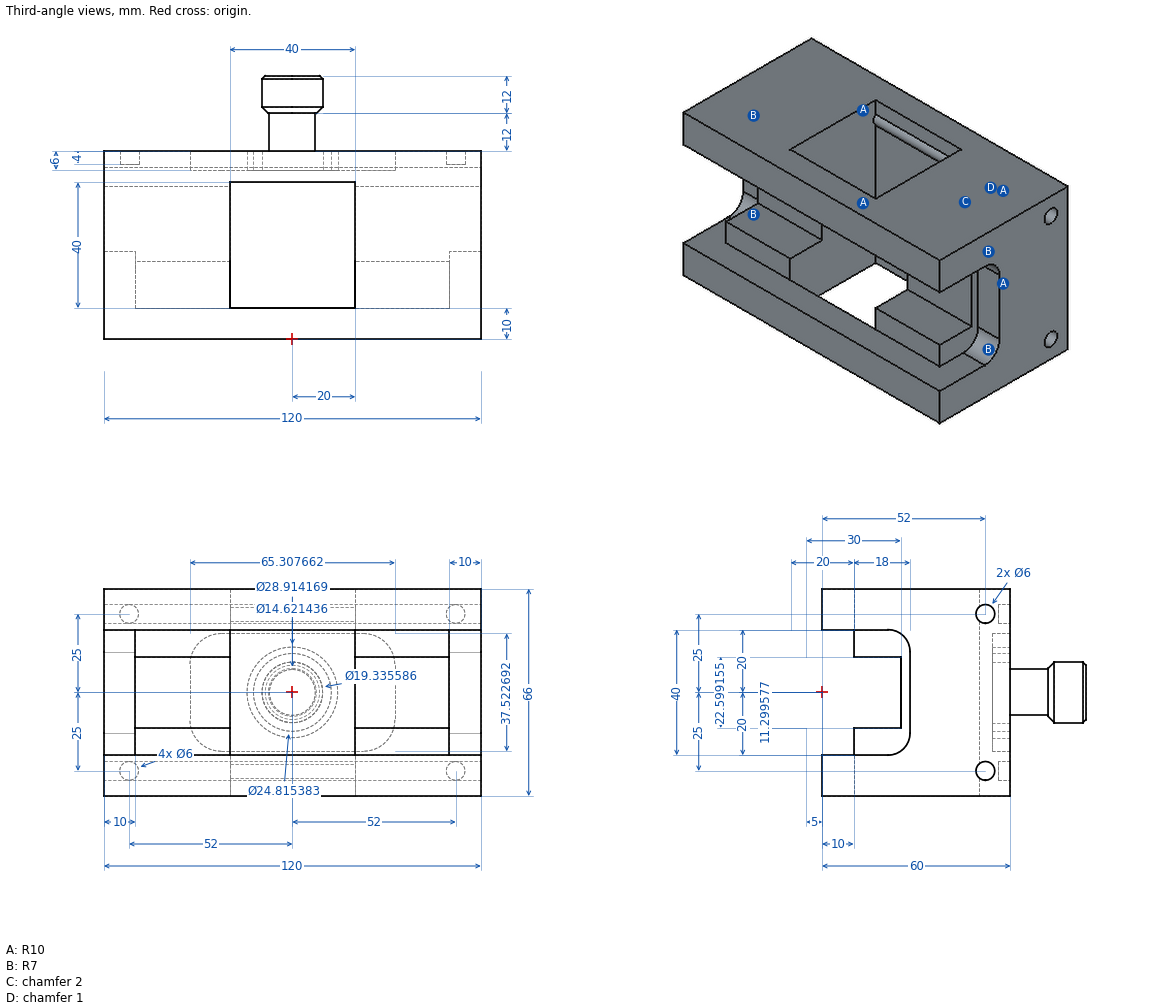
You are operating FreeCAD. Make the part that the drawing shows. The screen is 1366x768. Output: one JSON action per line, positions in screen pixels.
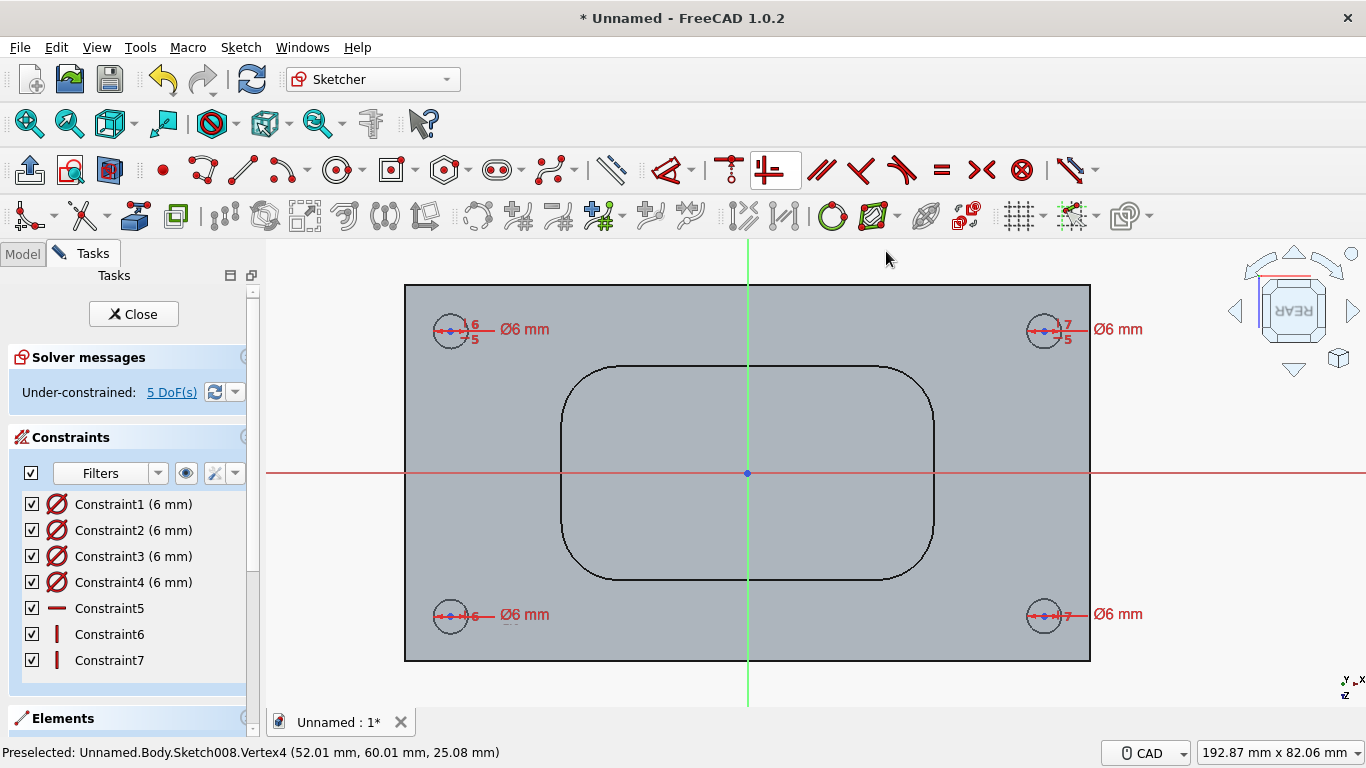
{"action": "left_click", "coordinate": [451, 617]}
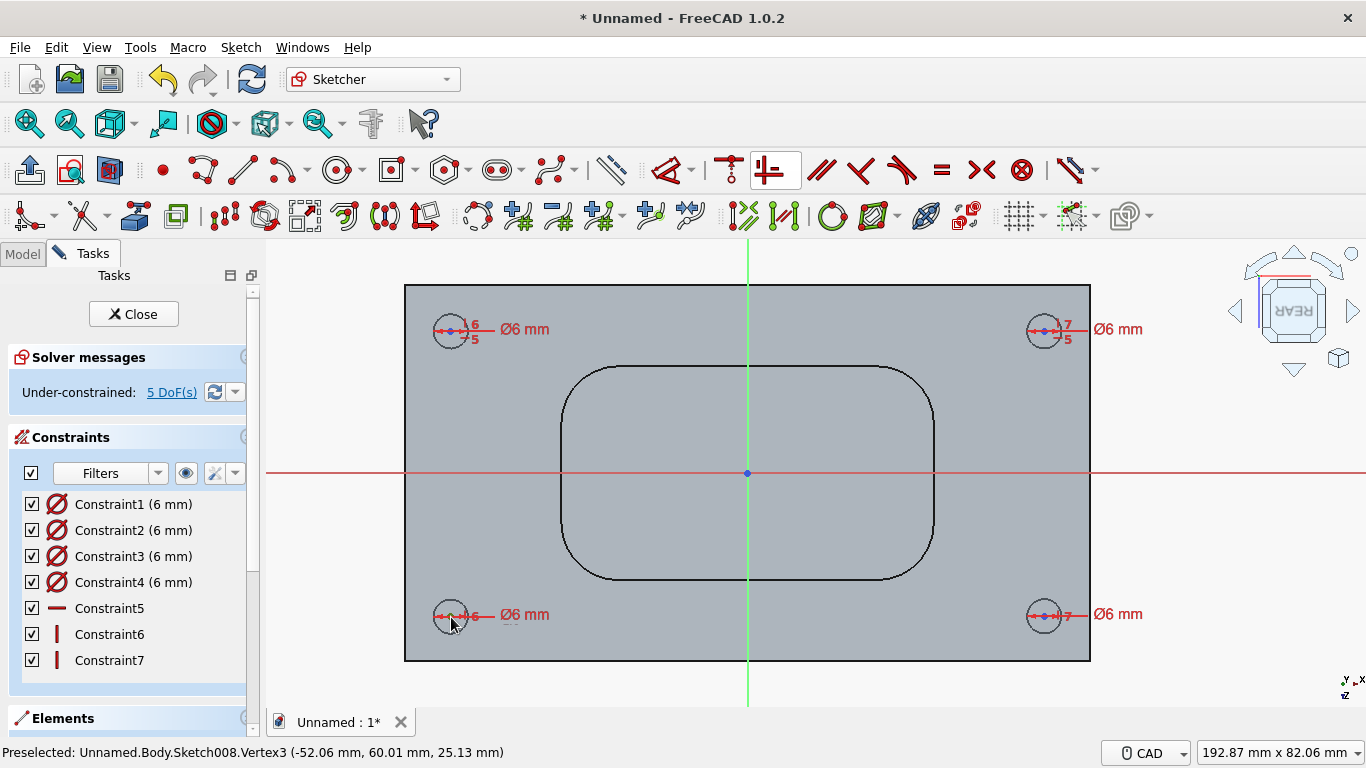
{"action": "left_click", "coordinate": [1044, 616]}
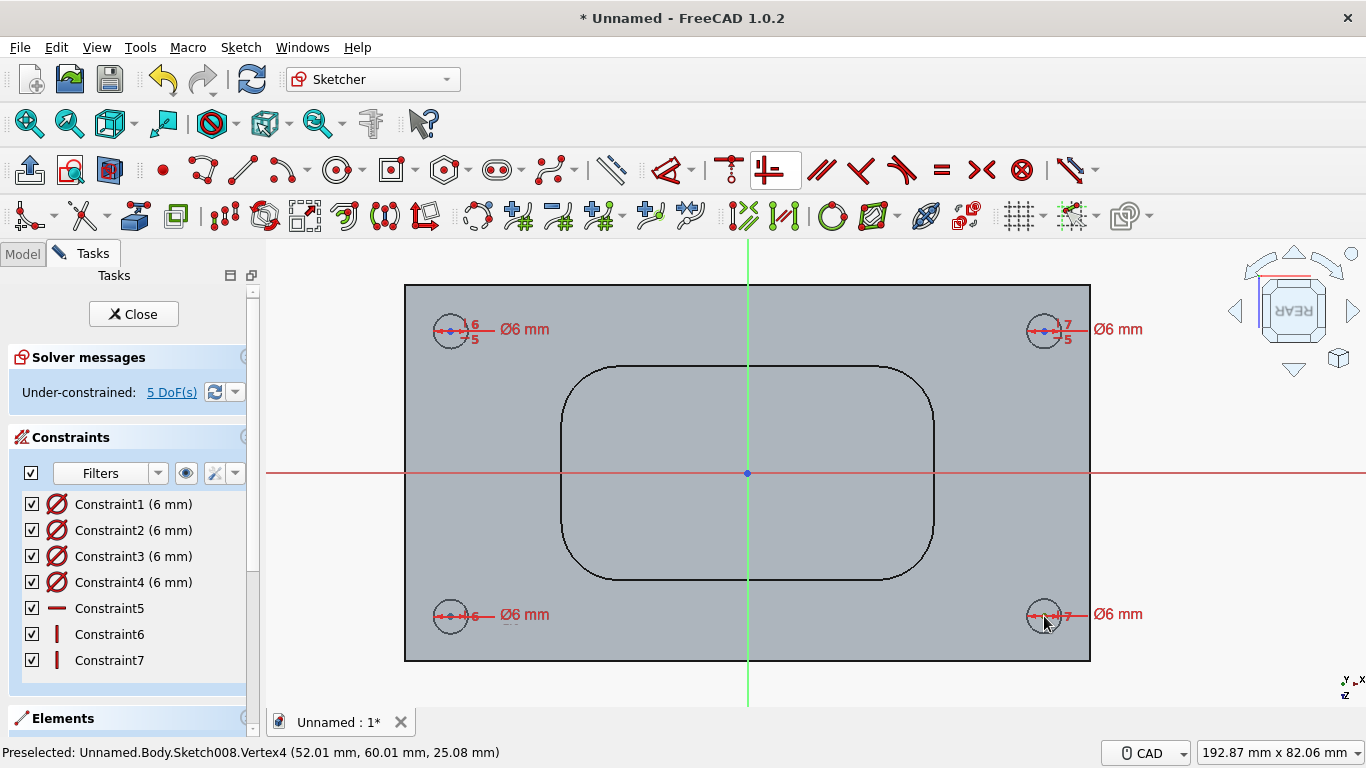
{"action": "key", "text": "h"}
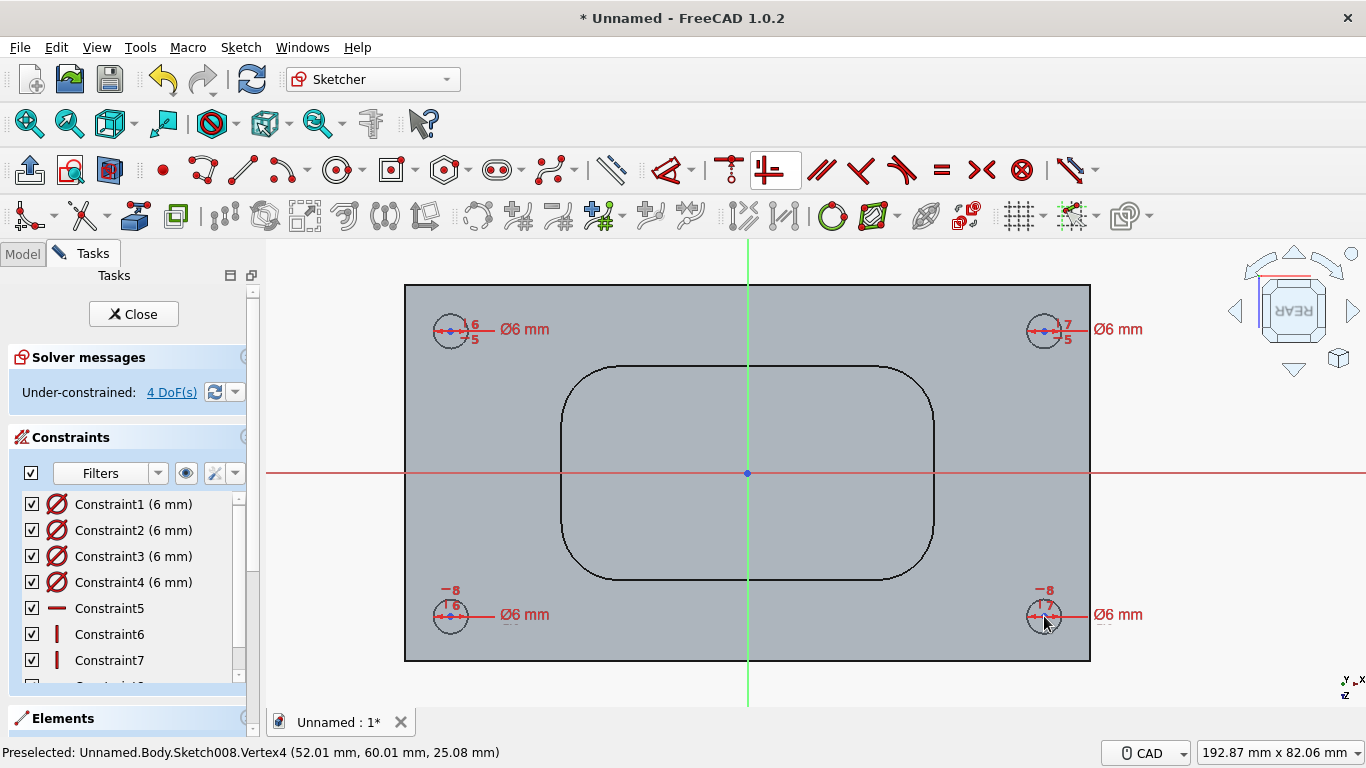
{"action": "left_click", "coordinate": [666, 170]}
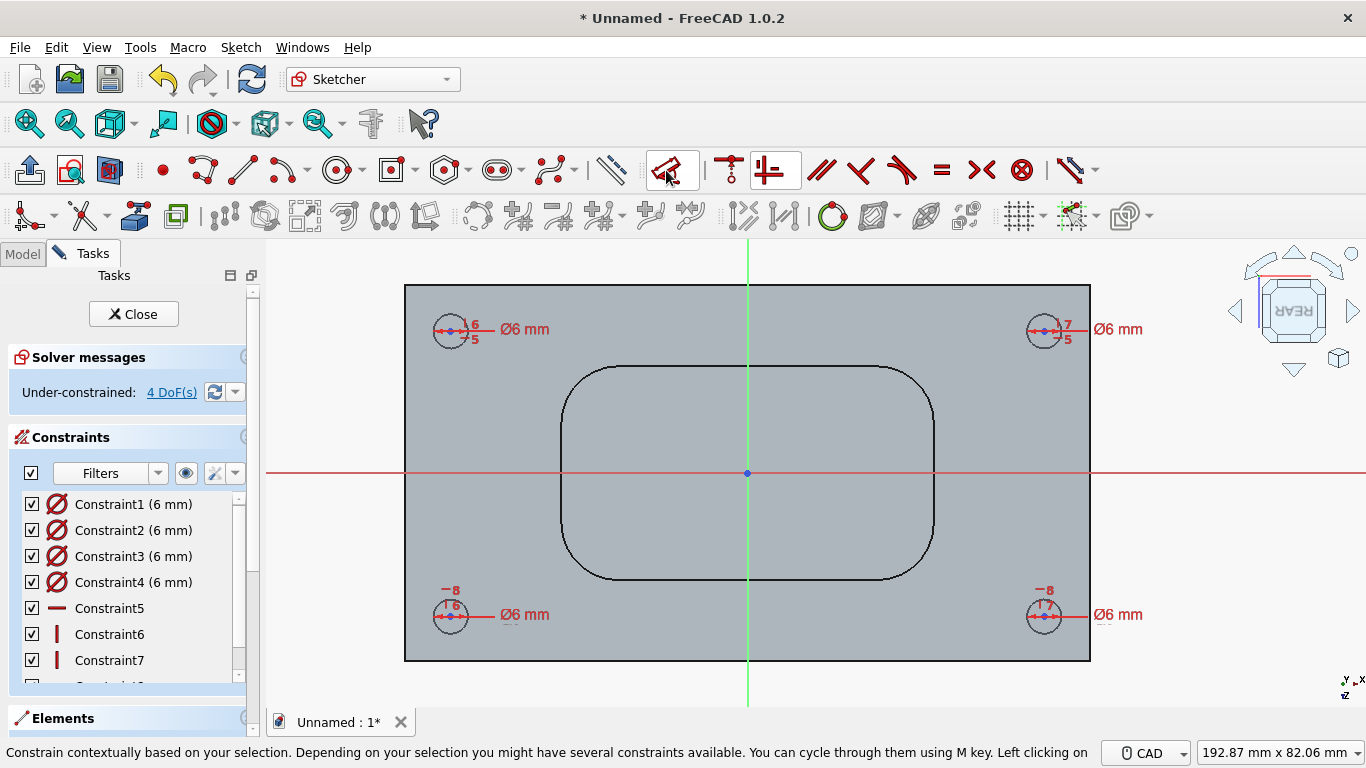
{"action": "left_click", "coordinate": [451, 331]}
{"action": "left_click", "coordinate": [599, 297]}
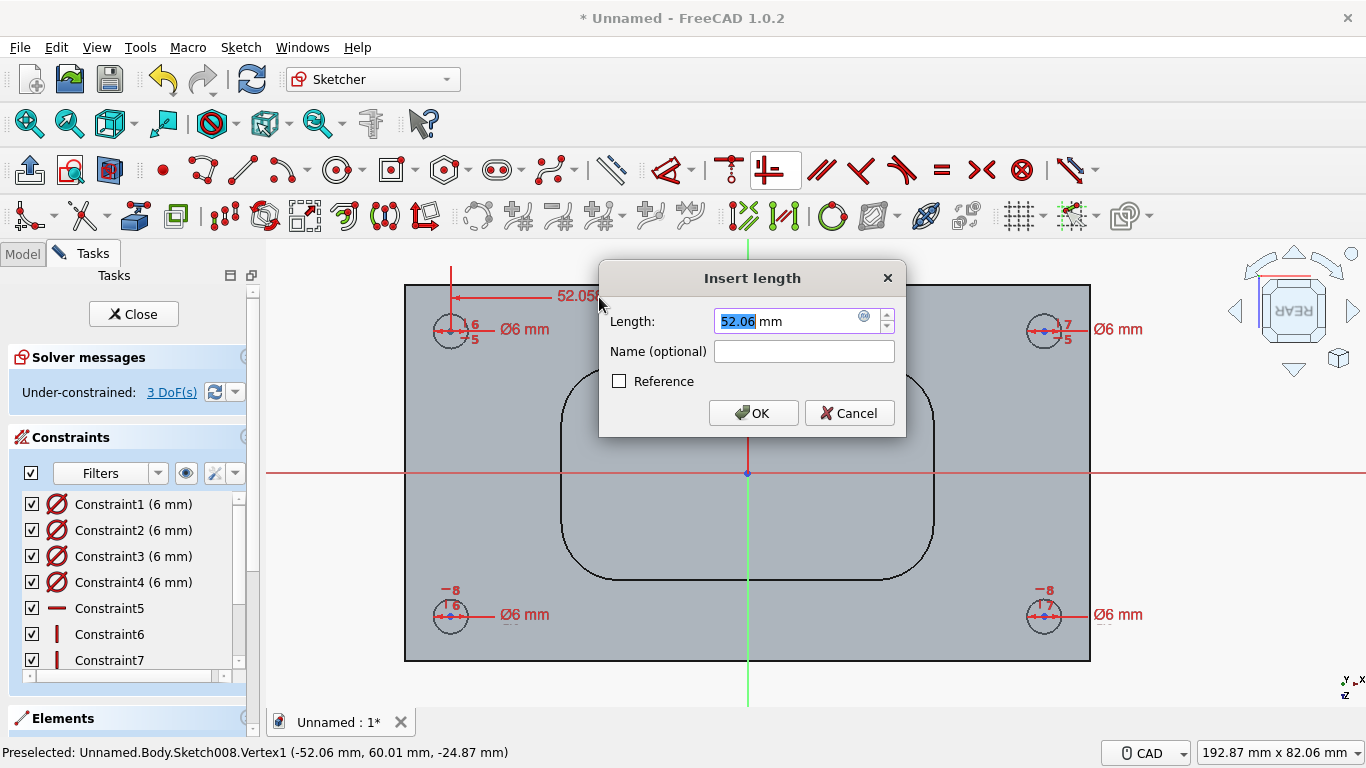
{"action": "type", "text": "52"}
{"action": "key", "text": "Return"}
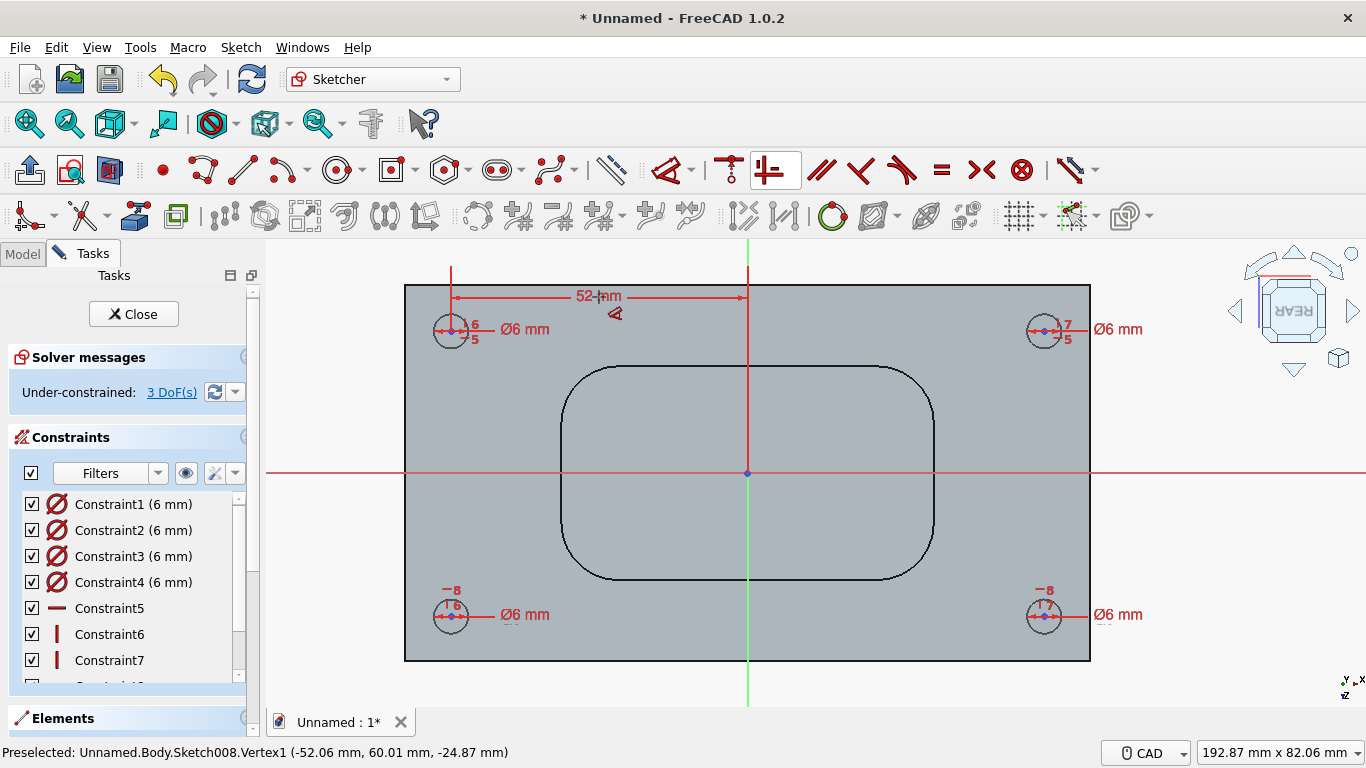
{"action": "left_click", "coordinate": [451, 331]}
{"action": "left_click", "coordinate": [417, 402]}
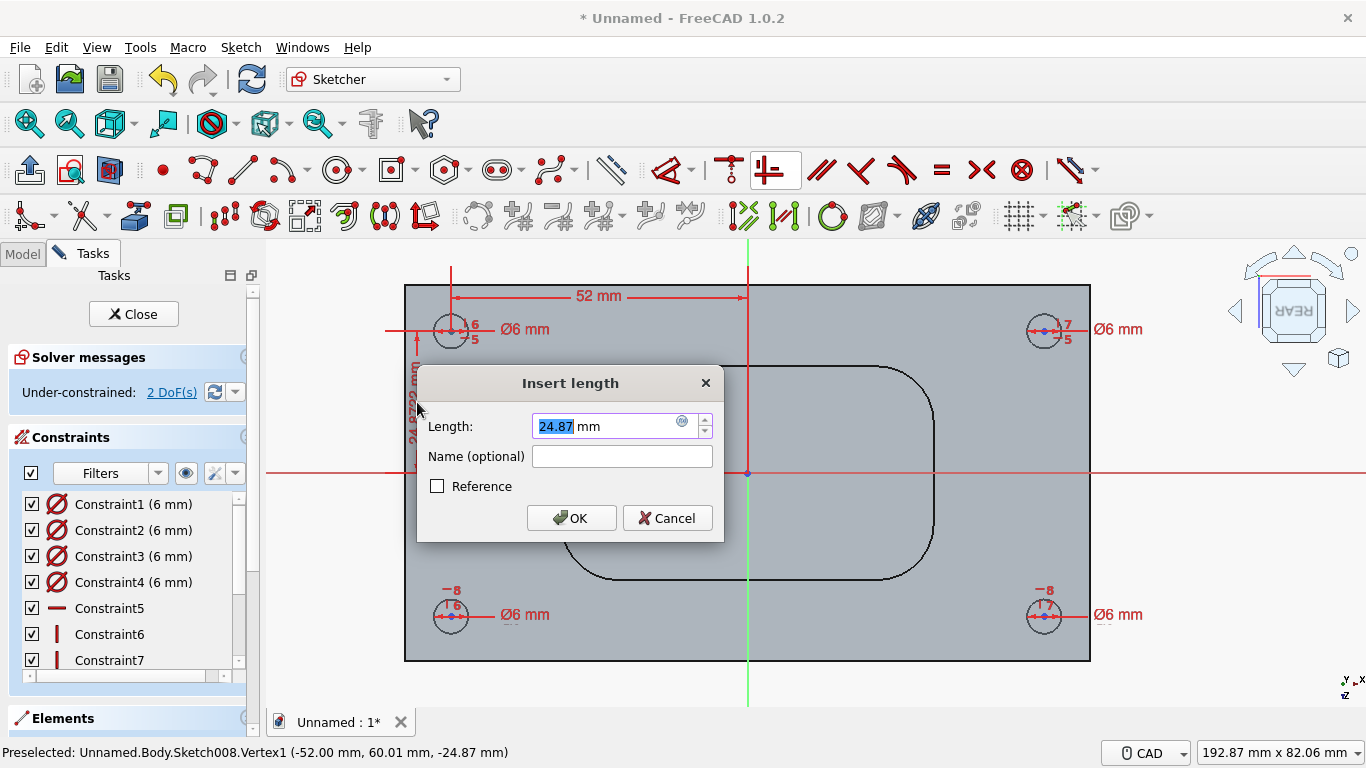
{"action": "type", "text": "25"}
{"action": "key", "text": "Return"}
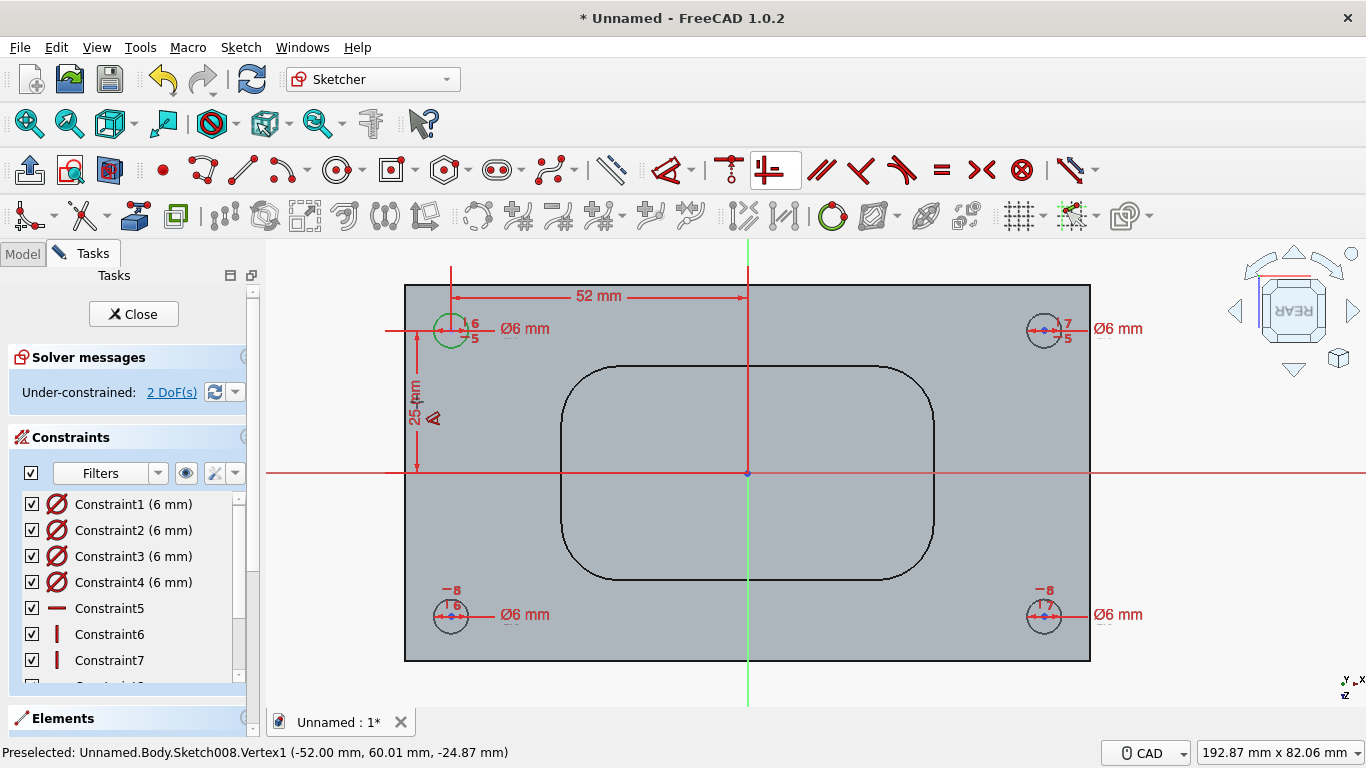
{"action": "left_click", "coordinate": [1044, 331]}
{"action": "left_click", "coordinate": [896, 297]}